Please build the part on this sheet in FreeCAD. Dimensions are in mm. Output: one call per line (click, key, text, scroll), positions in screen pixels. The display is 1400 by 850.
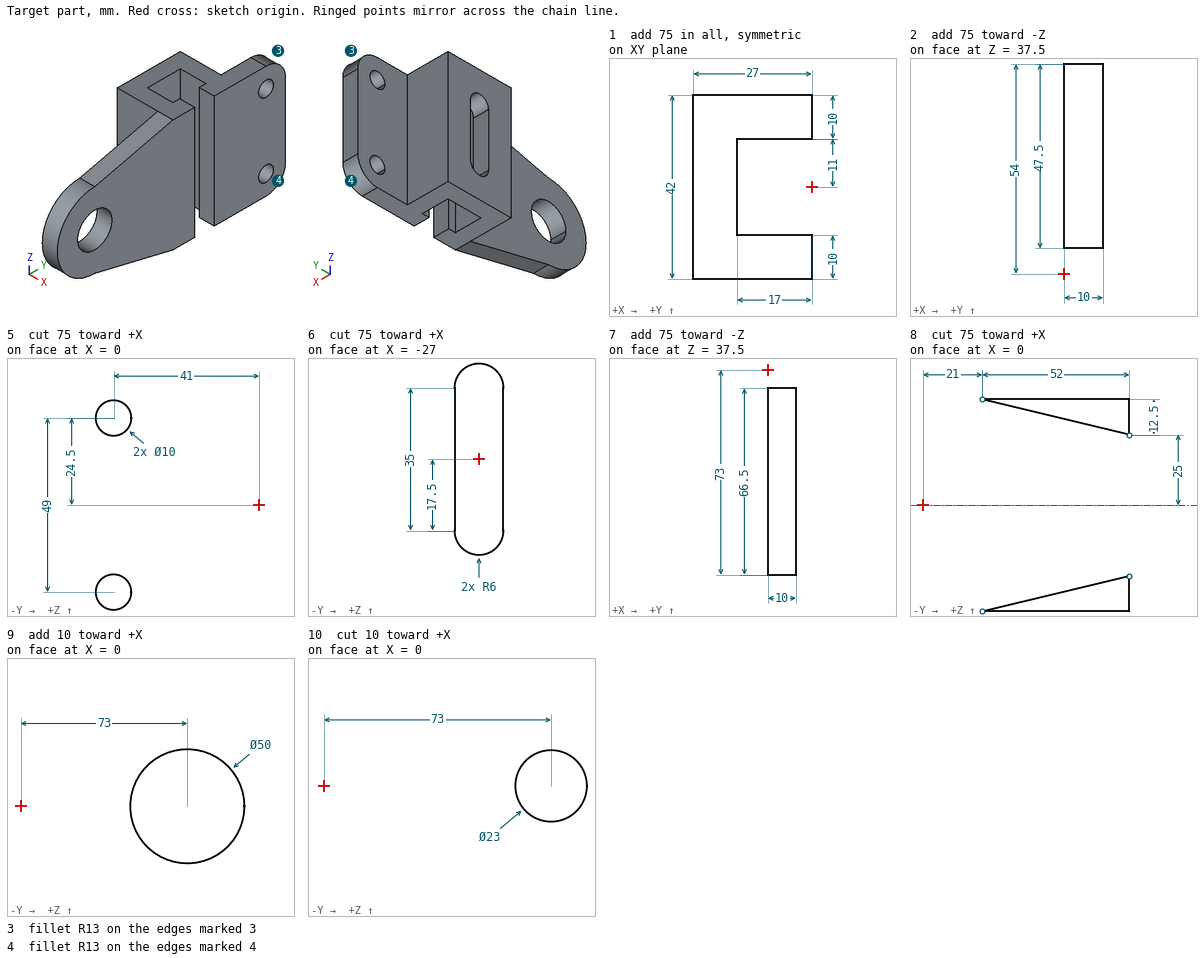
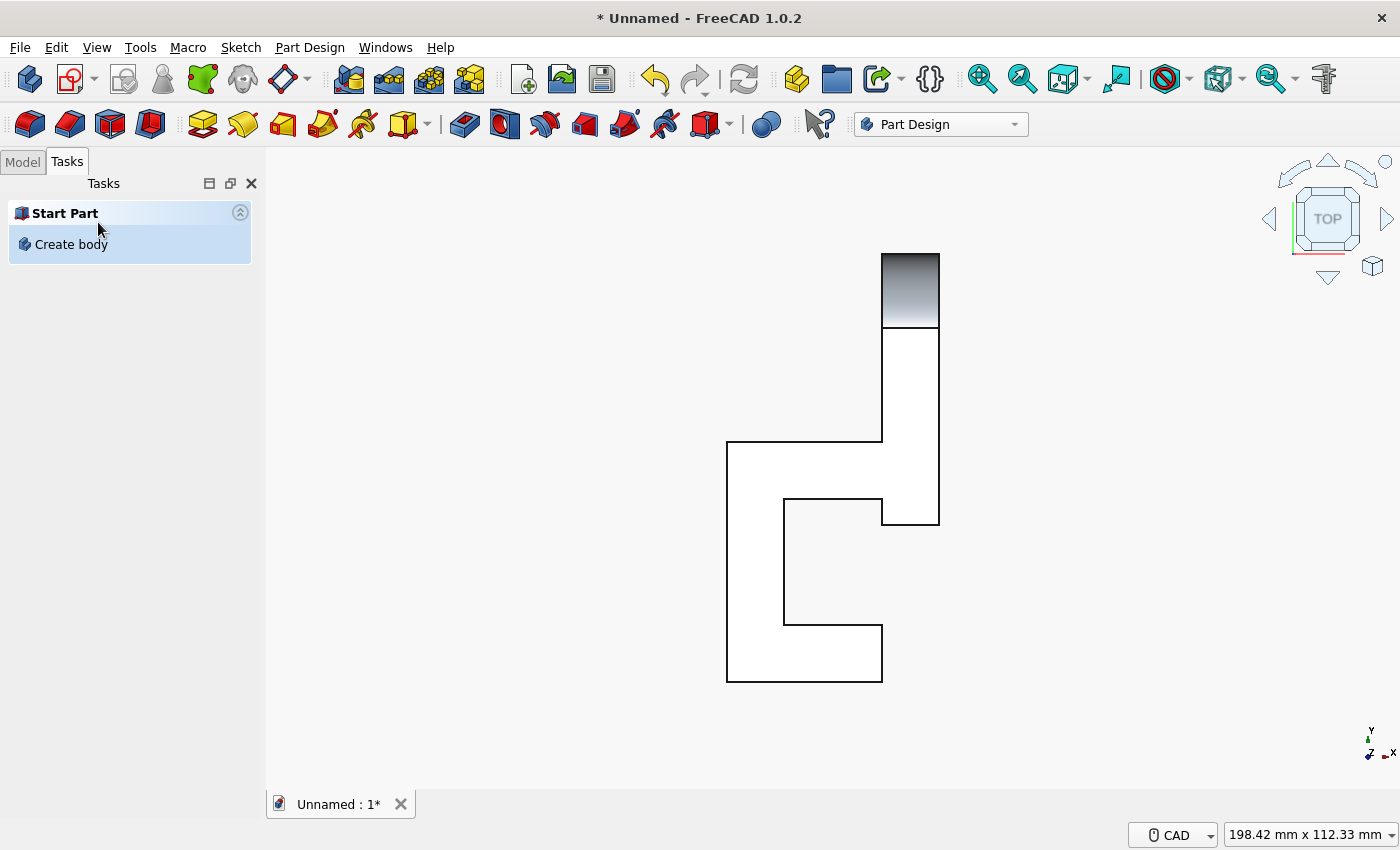
key(1)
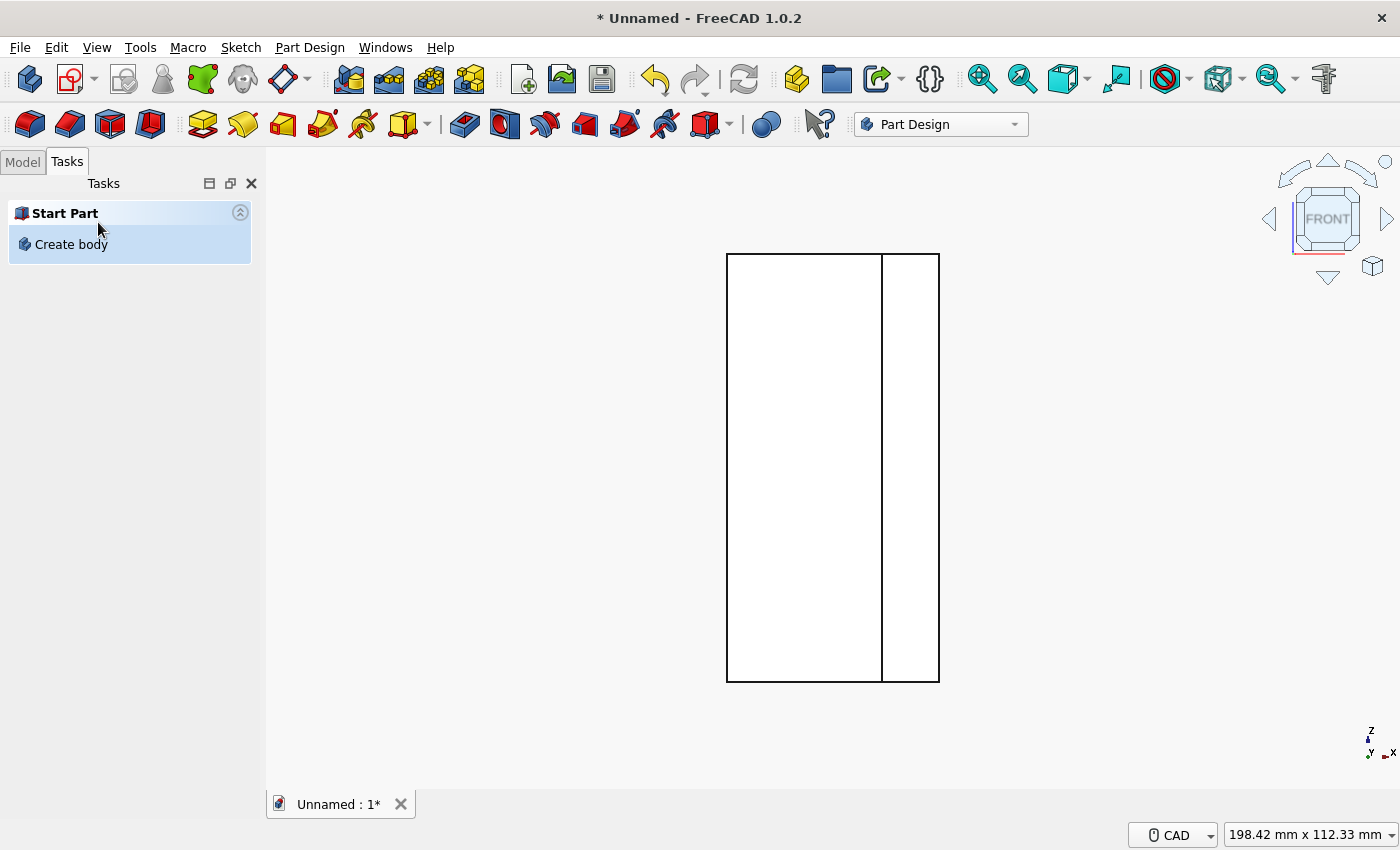
key(3)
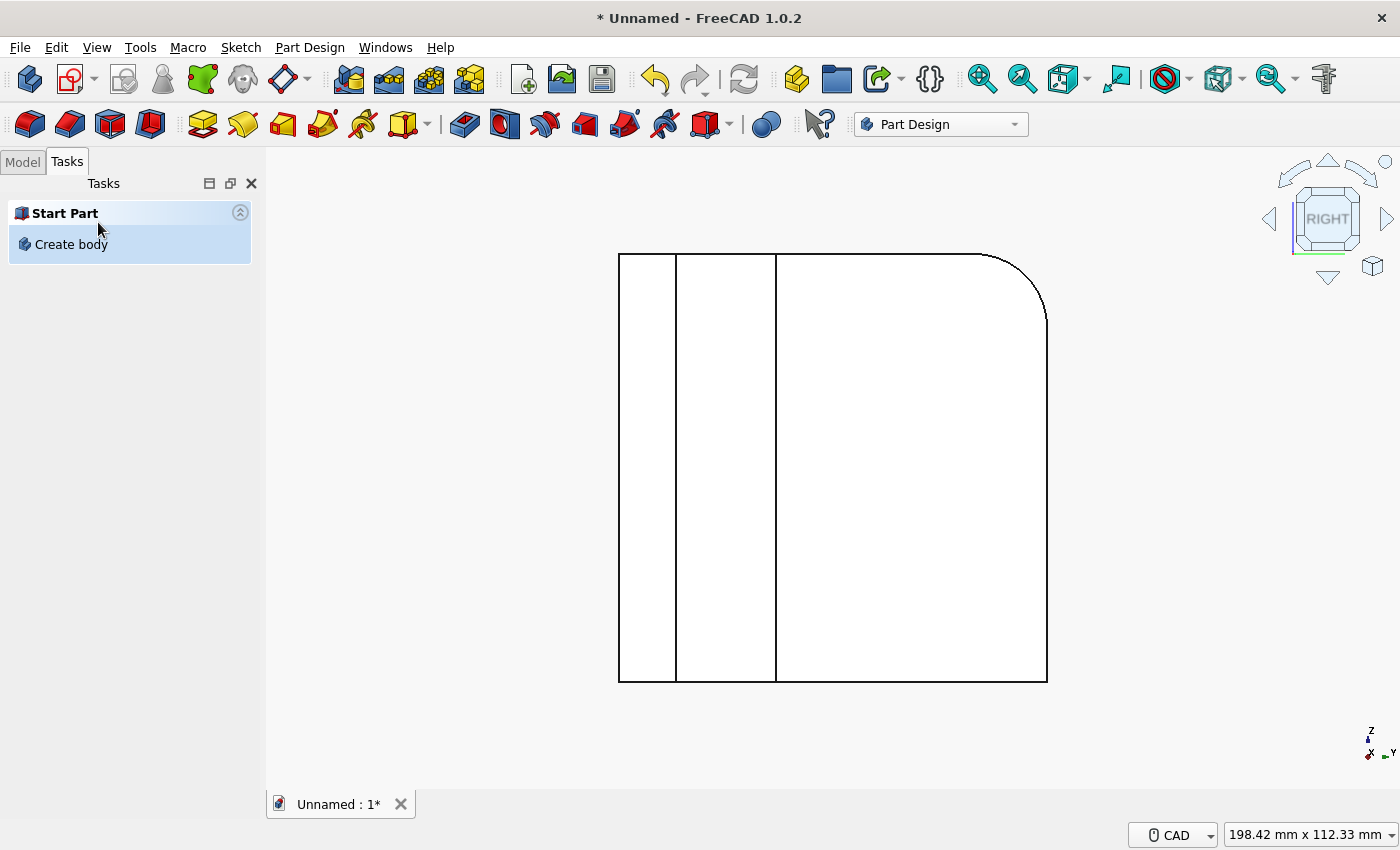
key(5)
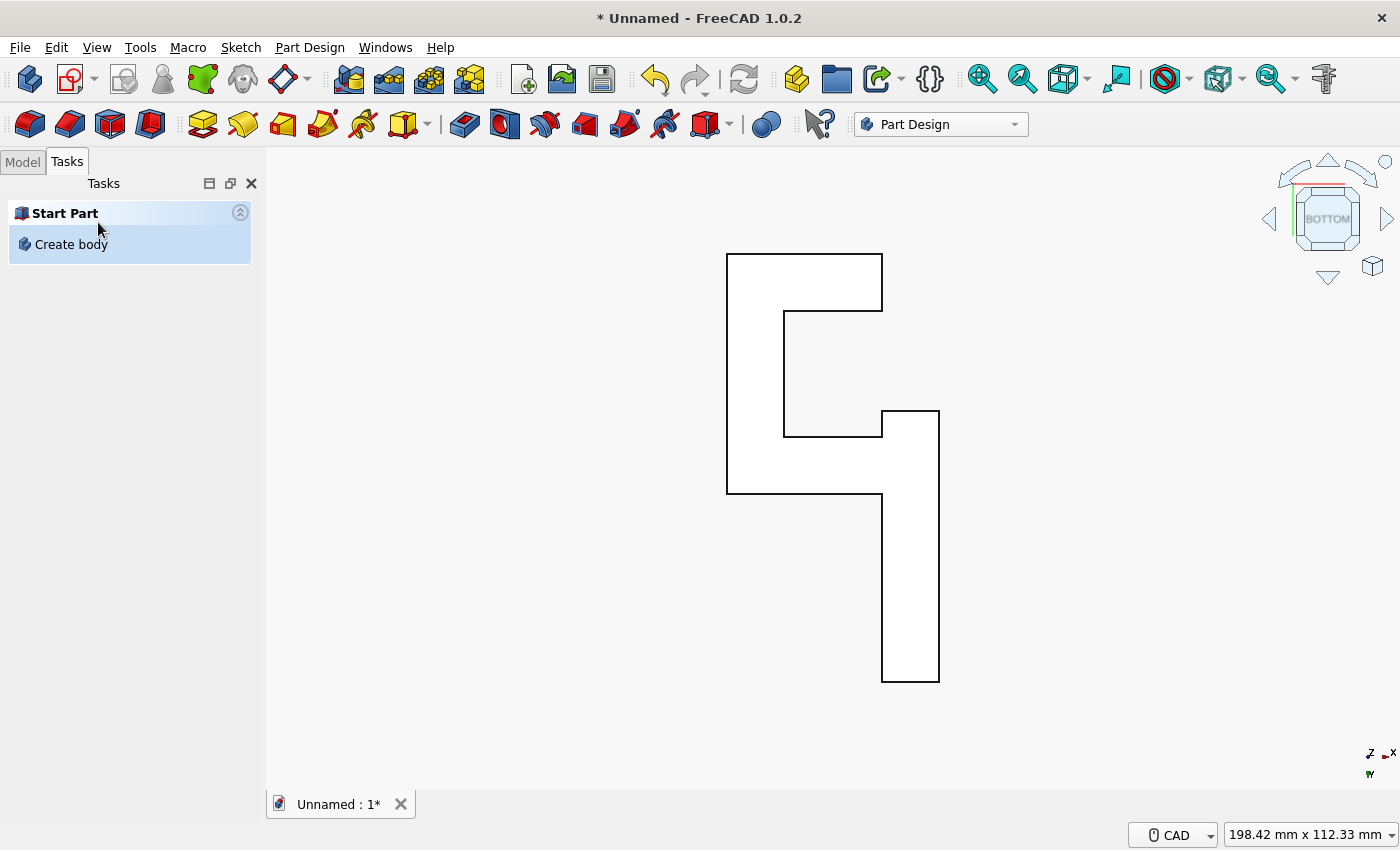
click(910, 681)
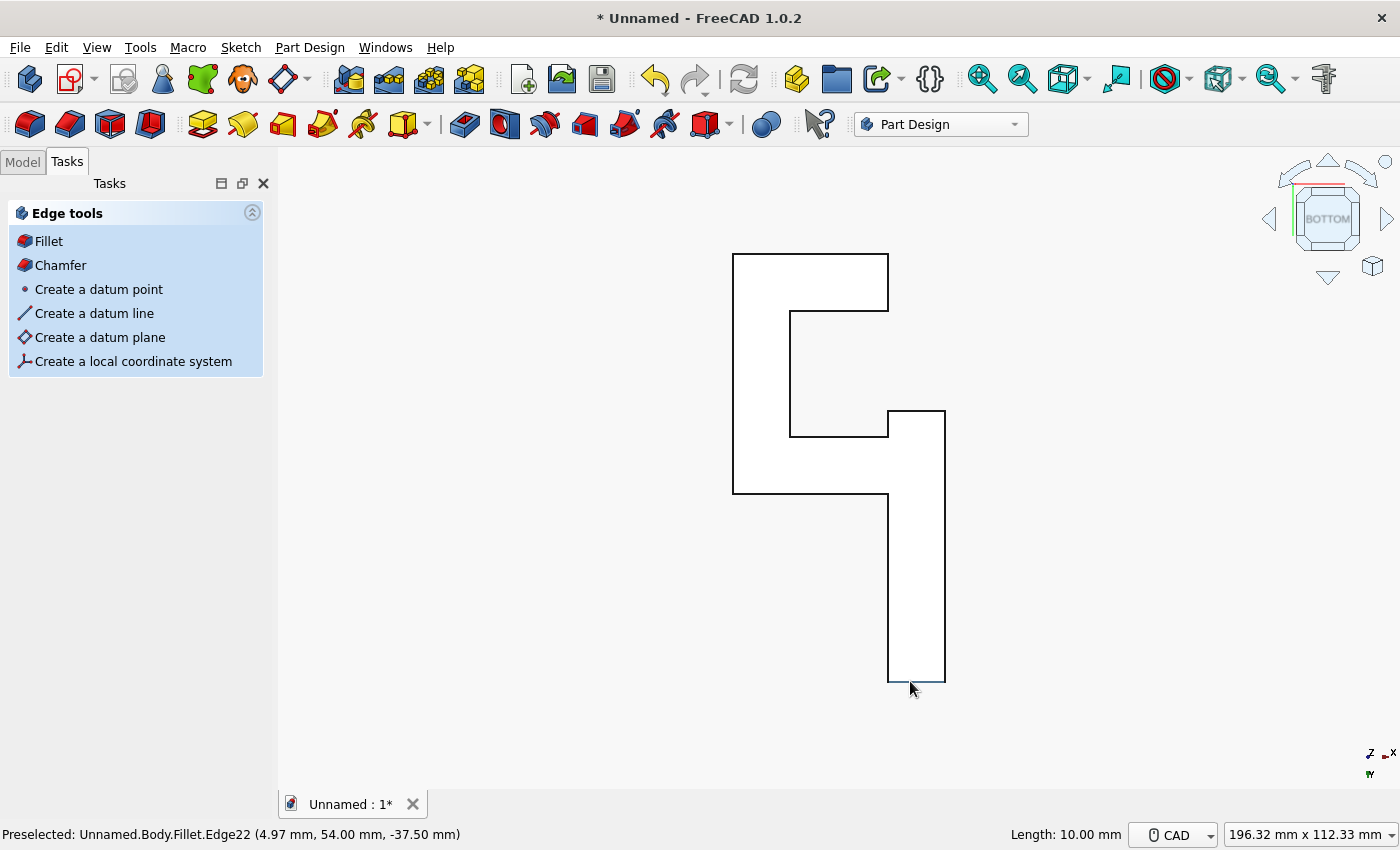
click(30, 124)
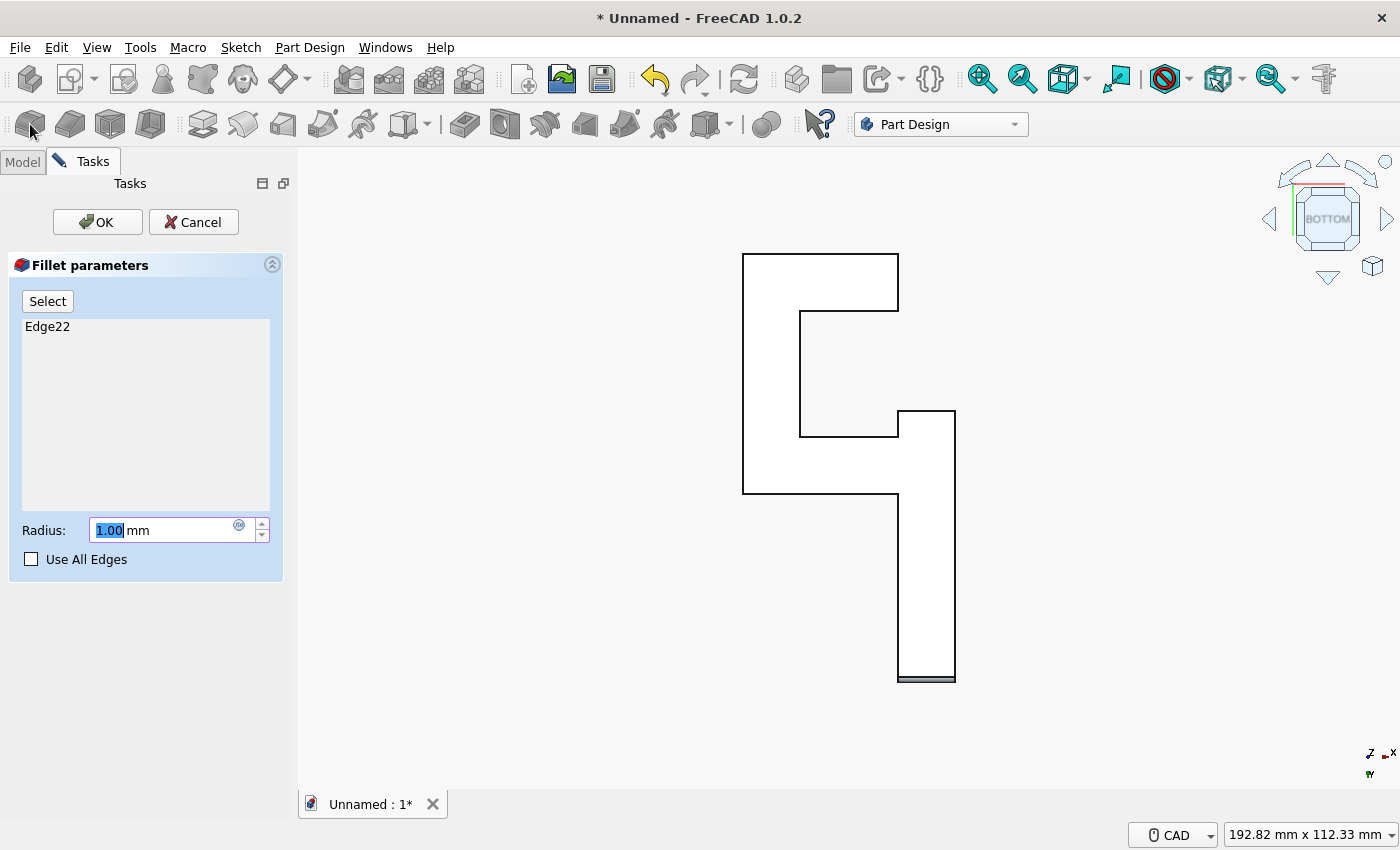
text(13)
key(Tab)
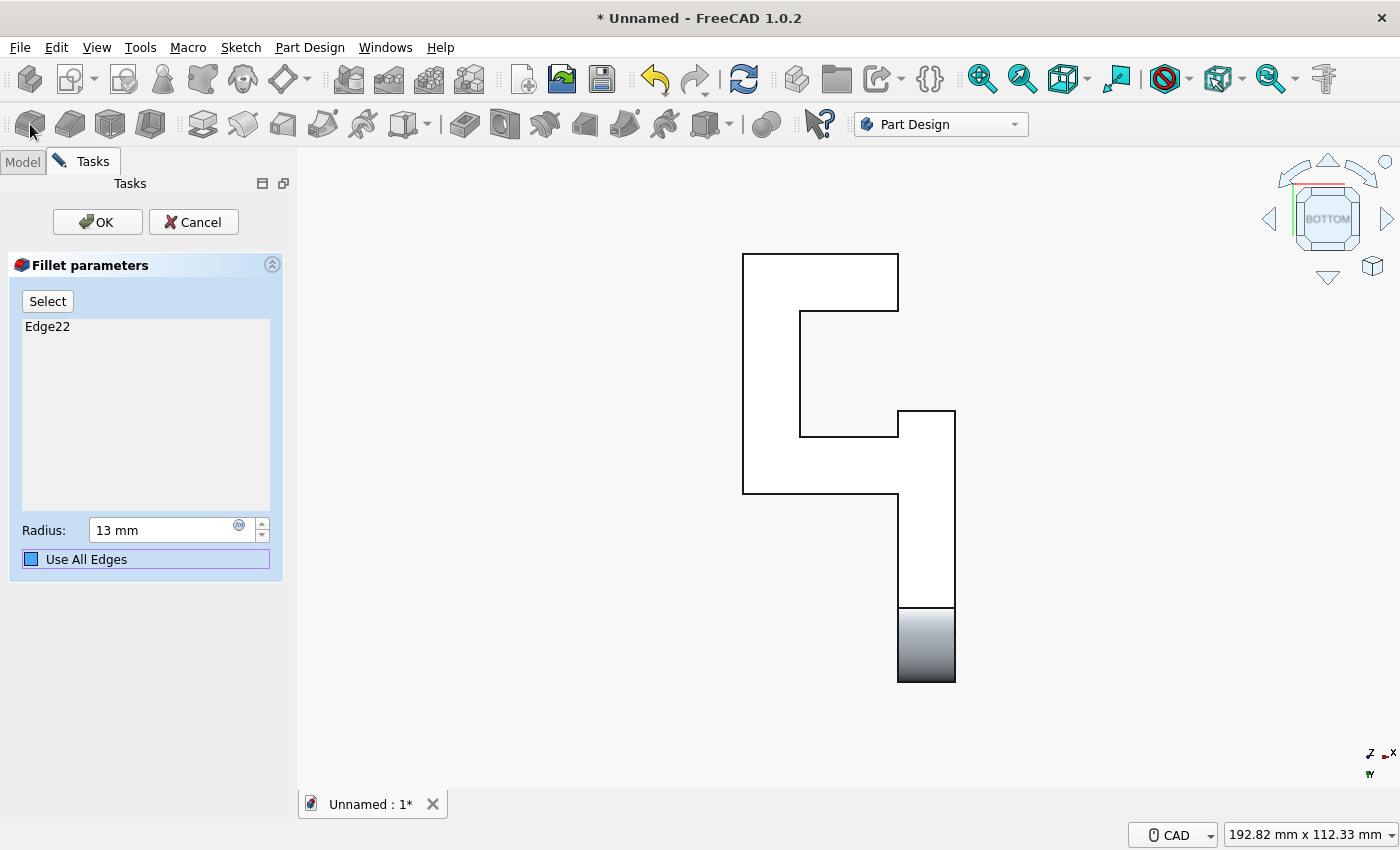
click(98, 222)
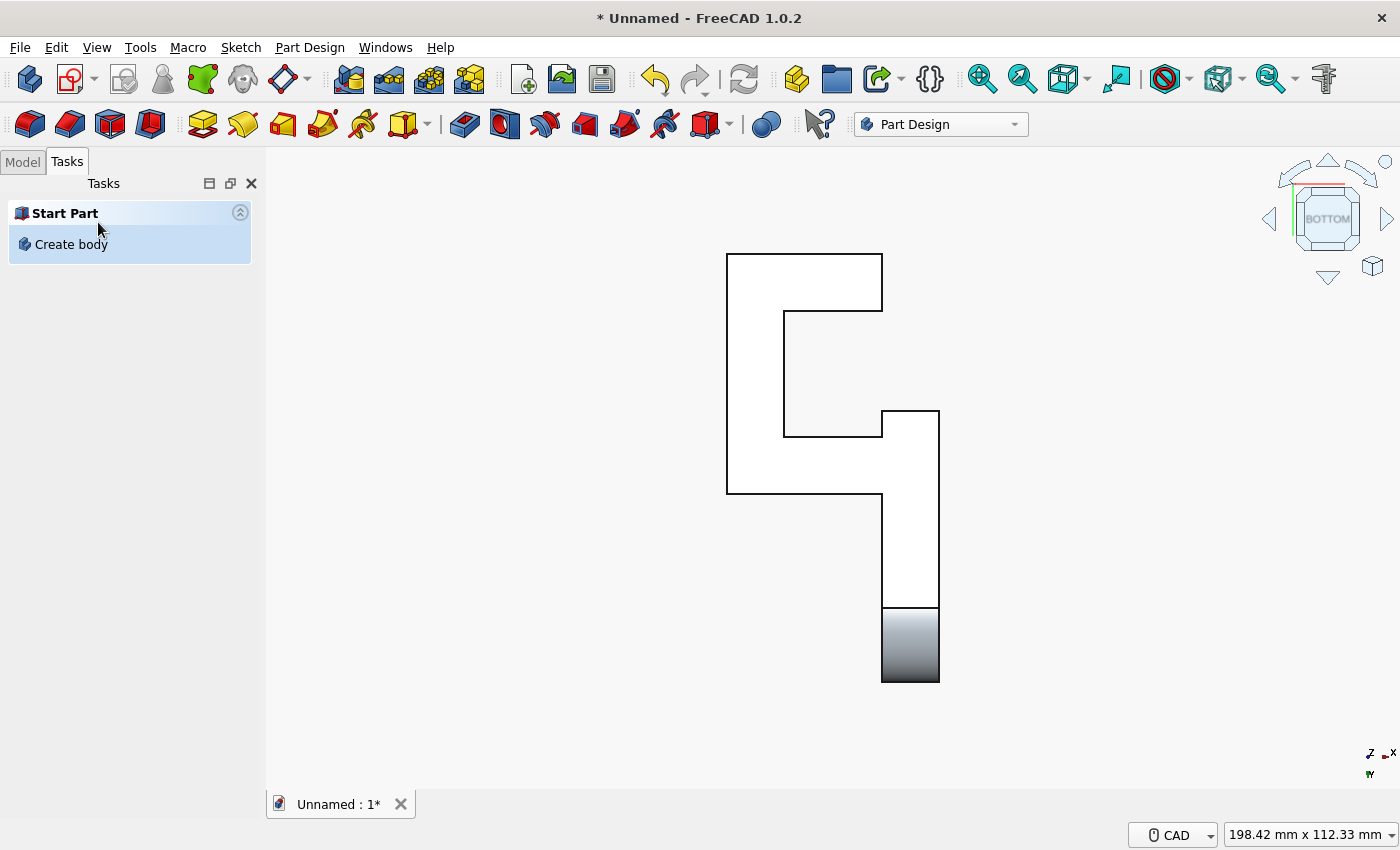
key(6)